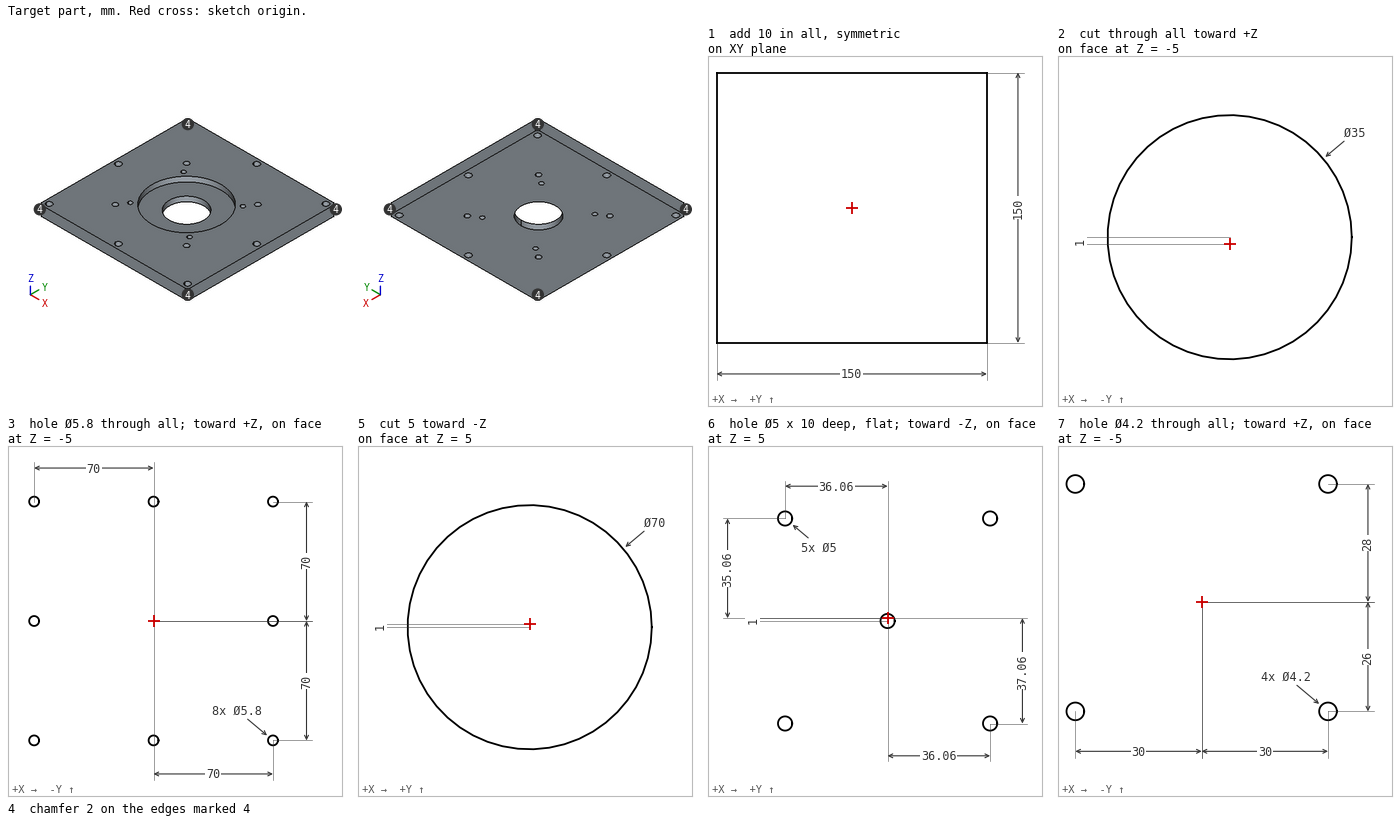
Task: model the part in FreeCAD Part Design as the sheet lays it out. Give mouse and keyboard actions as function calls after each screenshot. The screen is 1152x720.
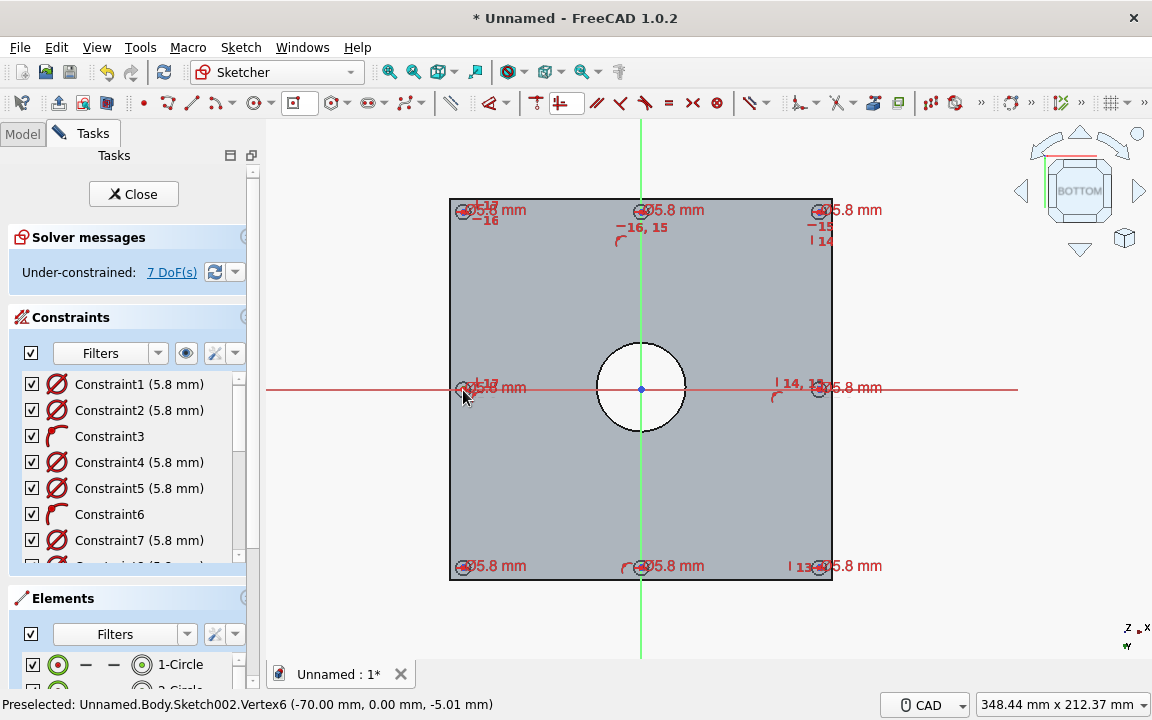
click(463, 568)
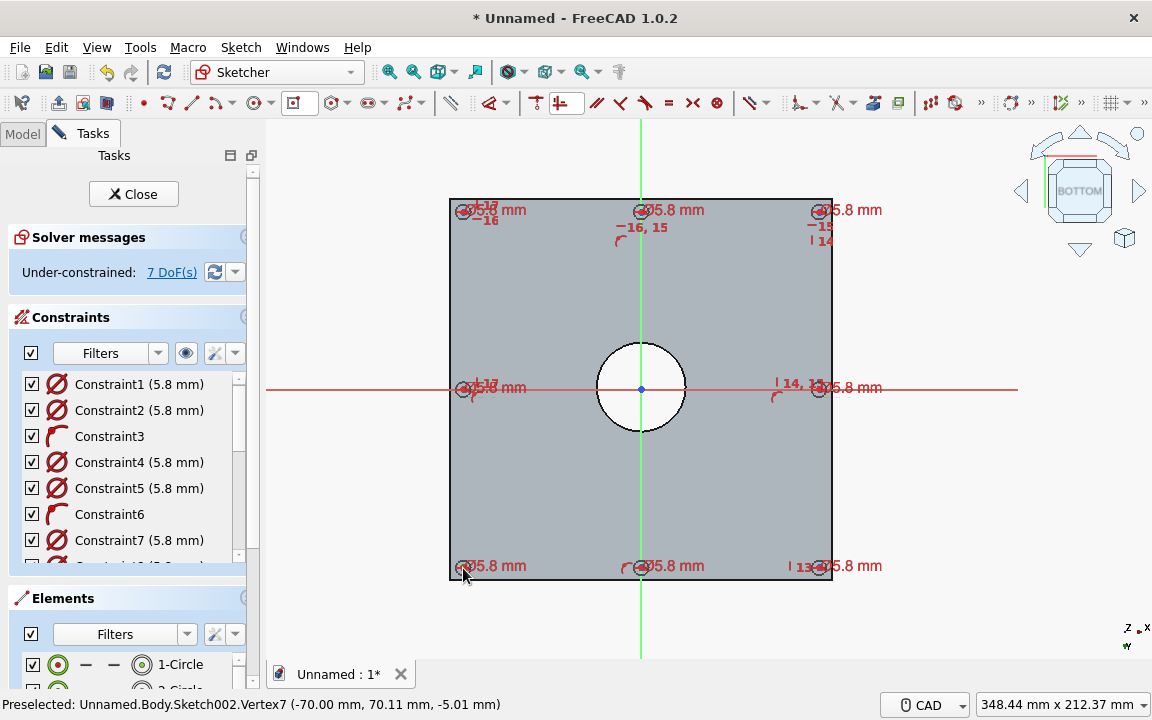
key(v)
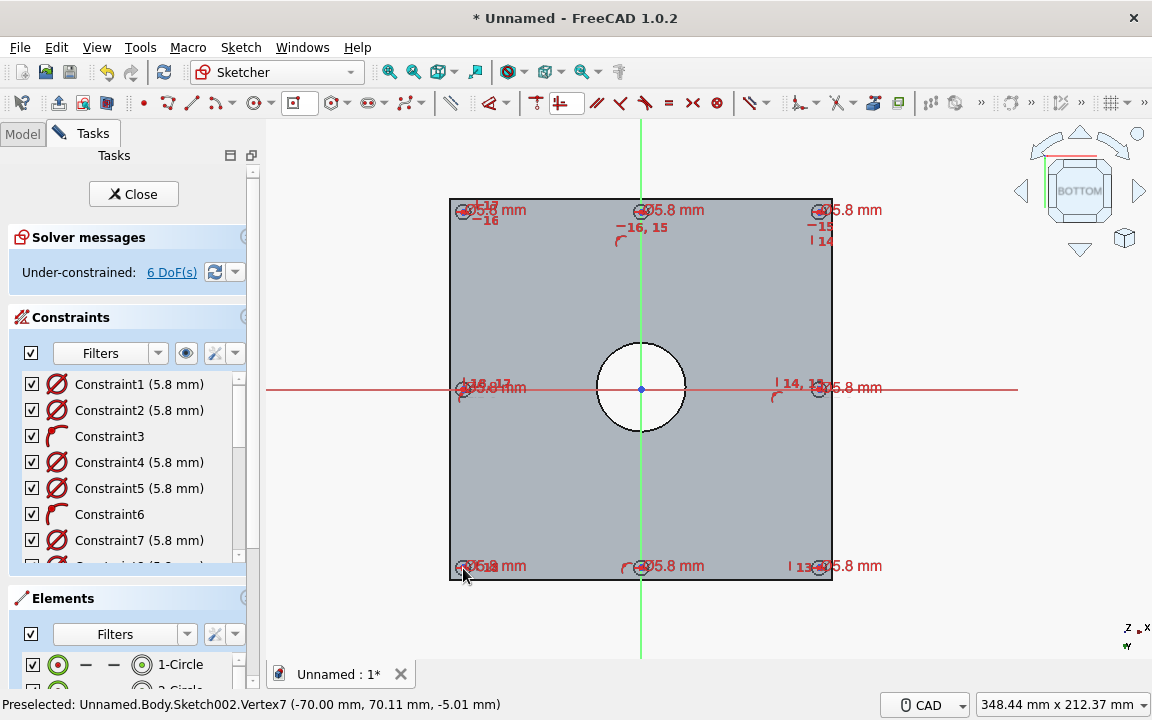
click(819, 568)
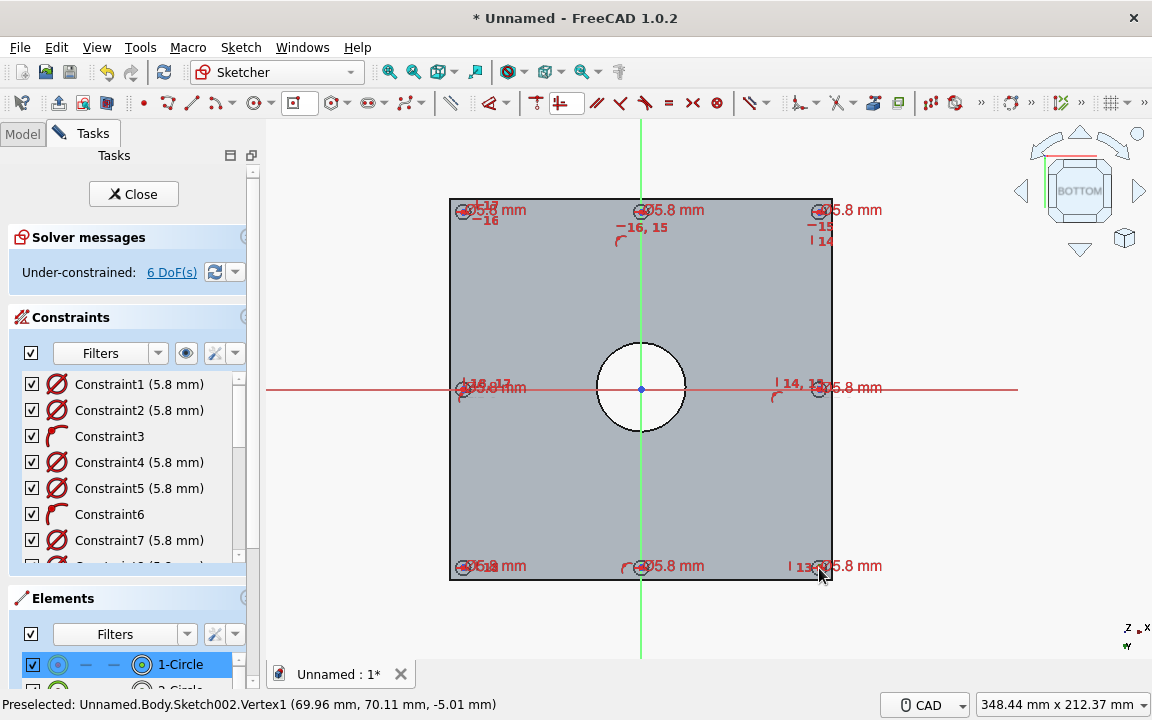
click(463, 568)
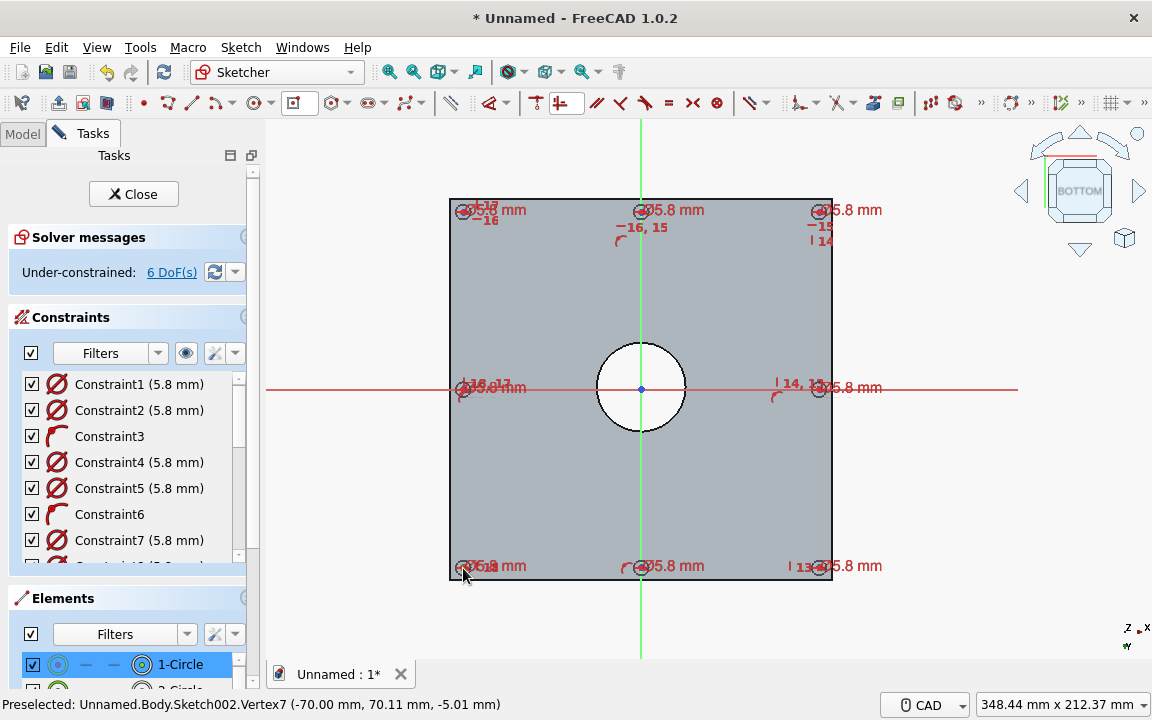
key(h)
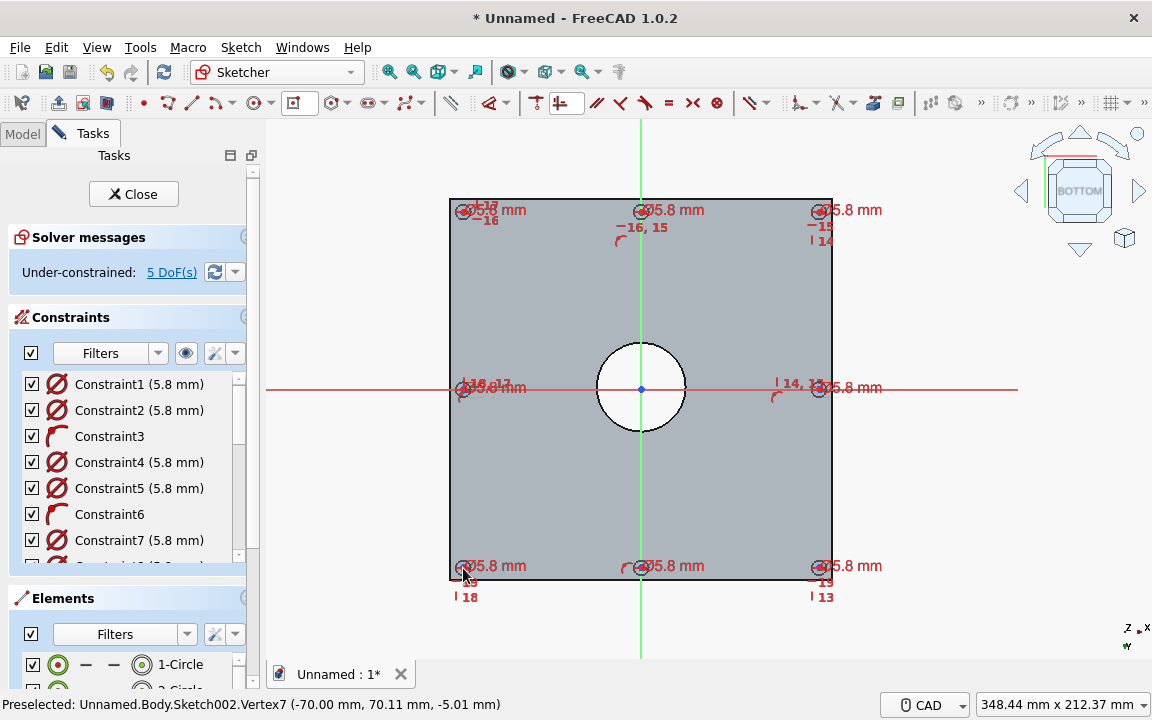
click(819, 568)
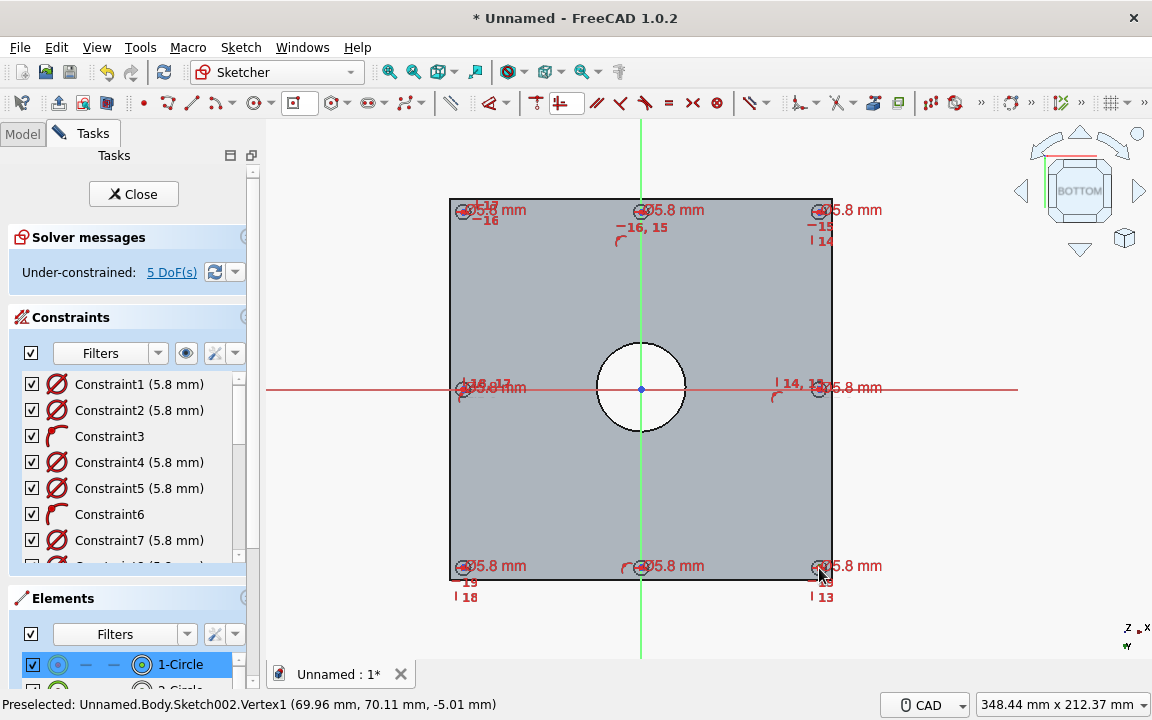
click(641, 568)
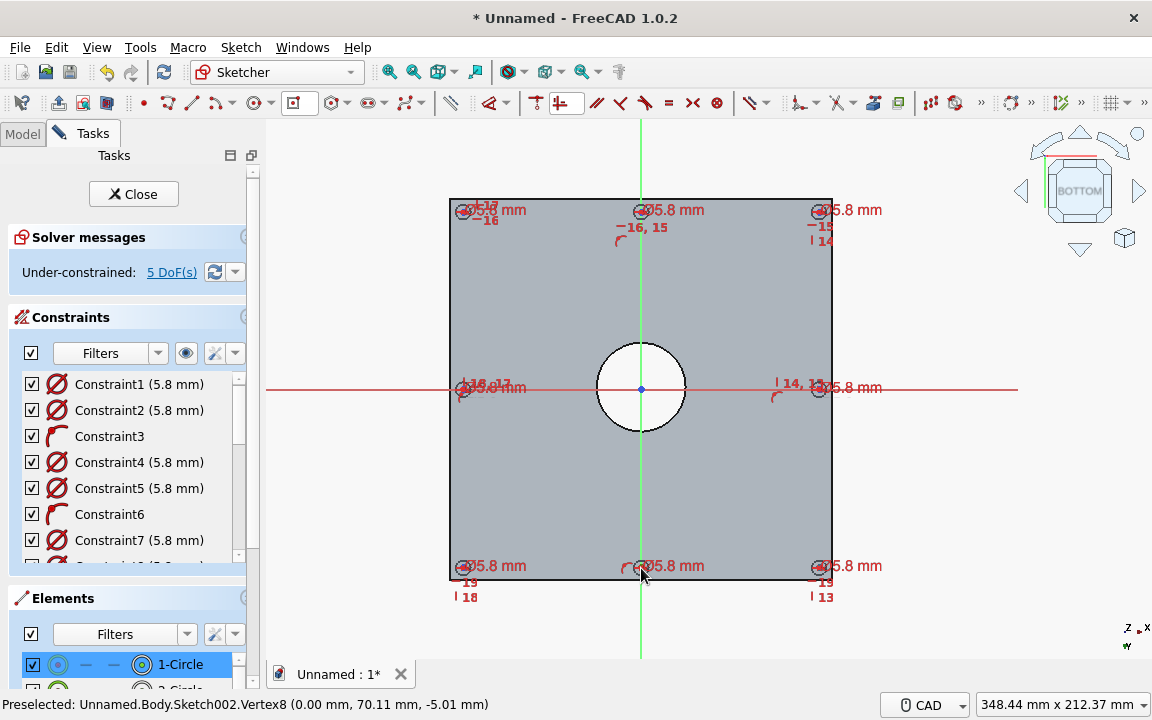
key(h)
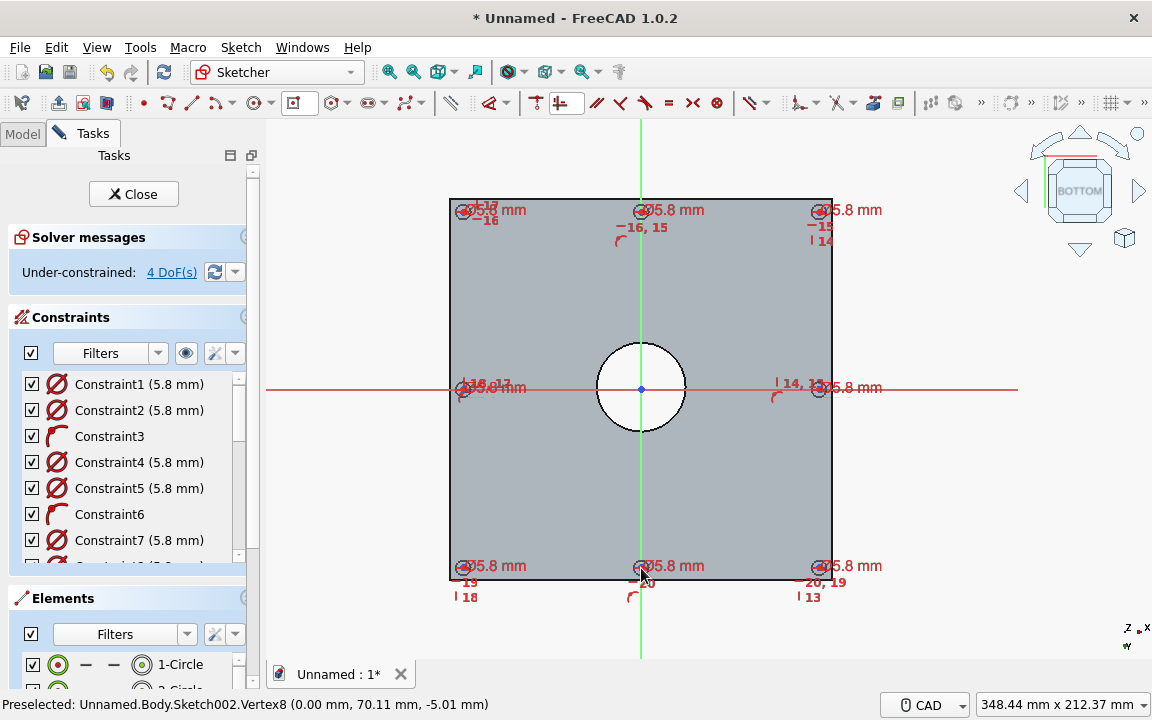
key(d)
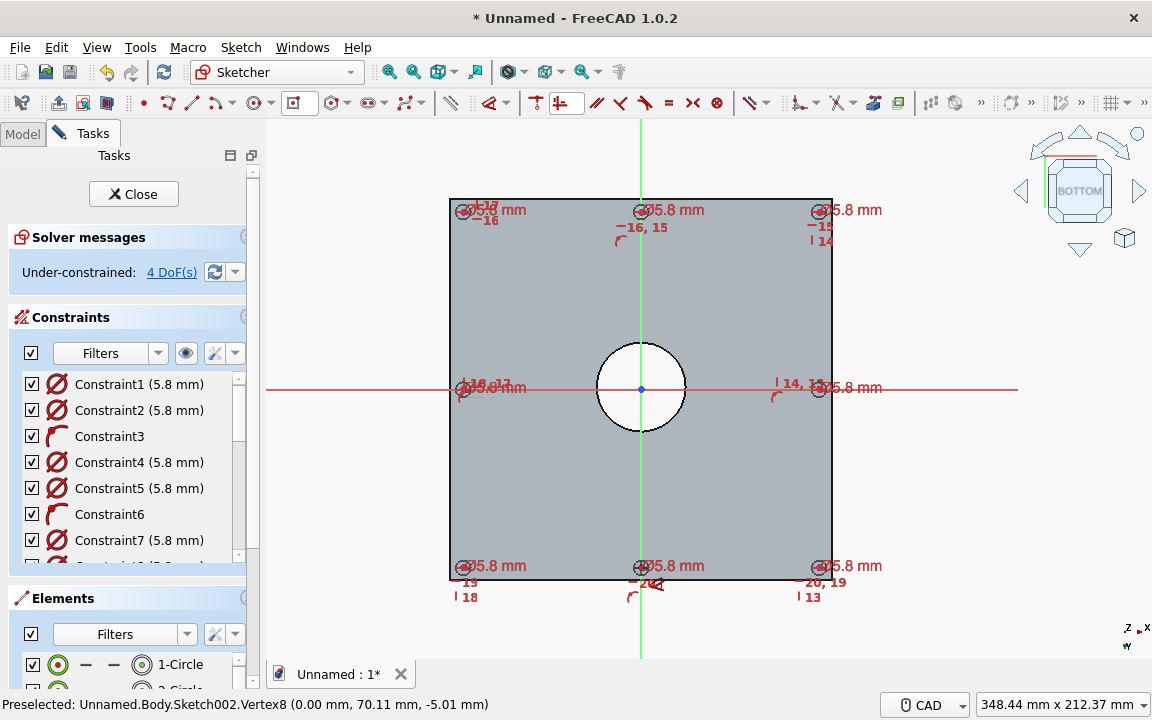
click(819, 568)
click(730, 602)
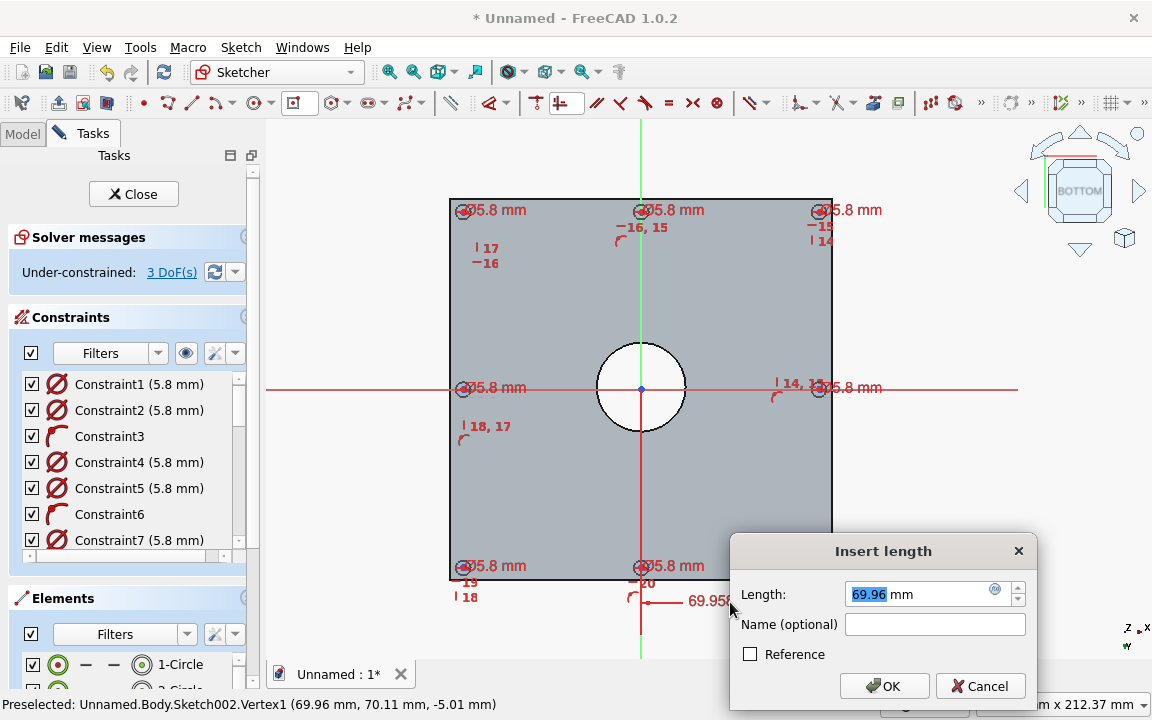
text(70)
key(Return)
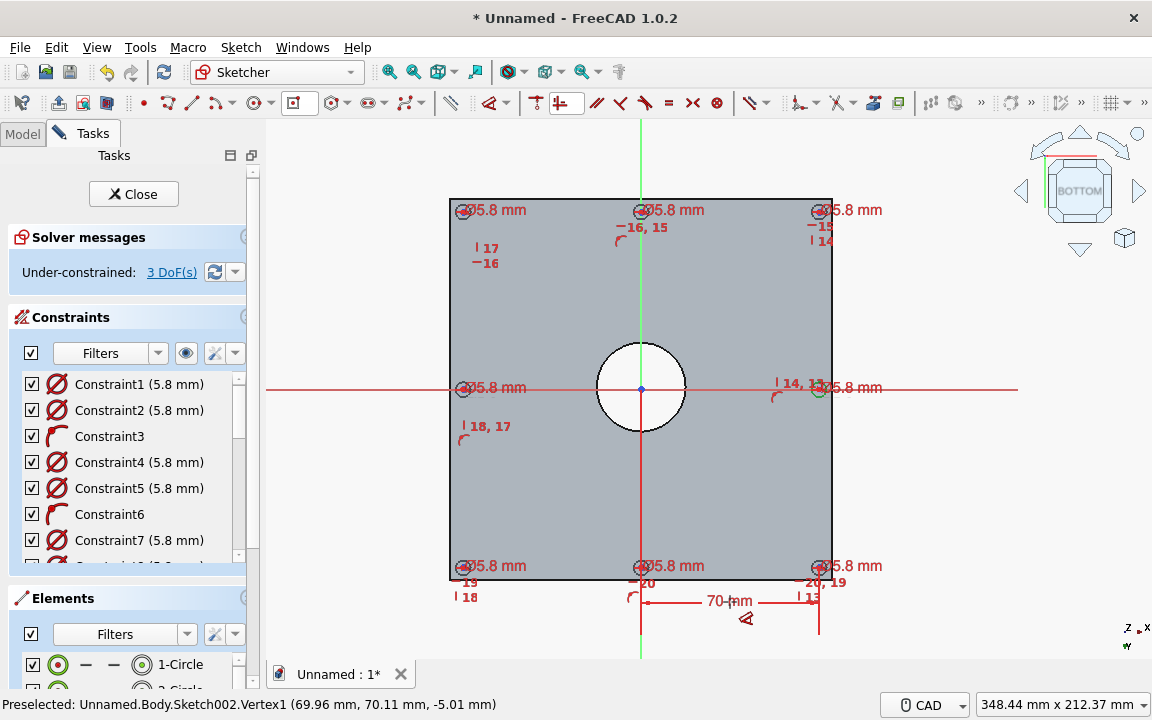
click(819, 568)
click(853, 479)